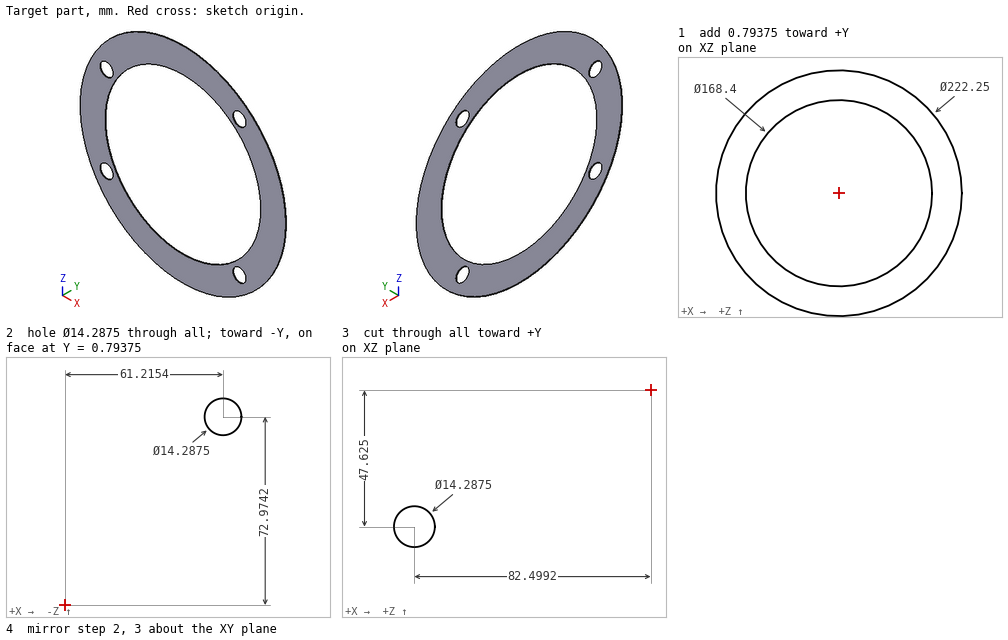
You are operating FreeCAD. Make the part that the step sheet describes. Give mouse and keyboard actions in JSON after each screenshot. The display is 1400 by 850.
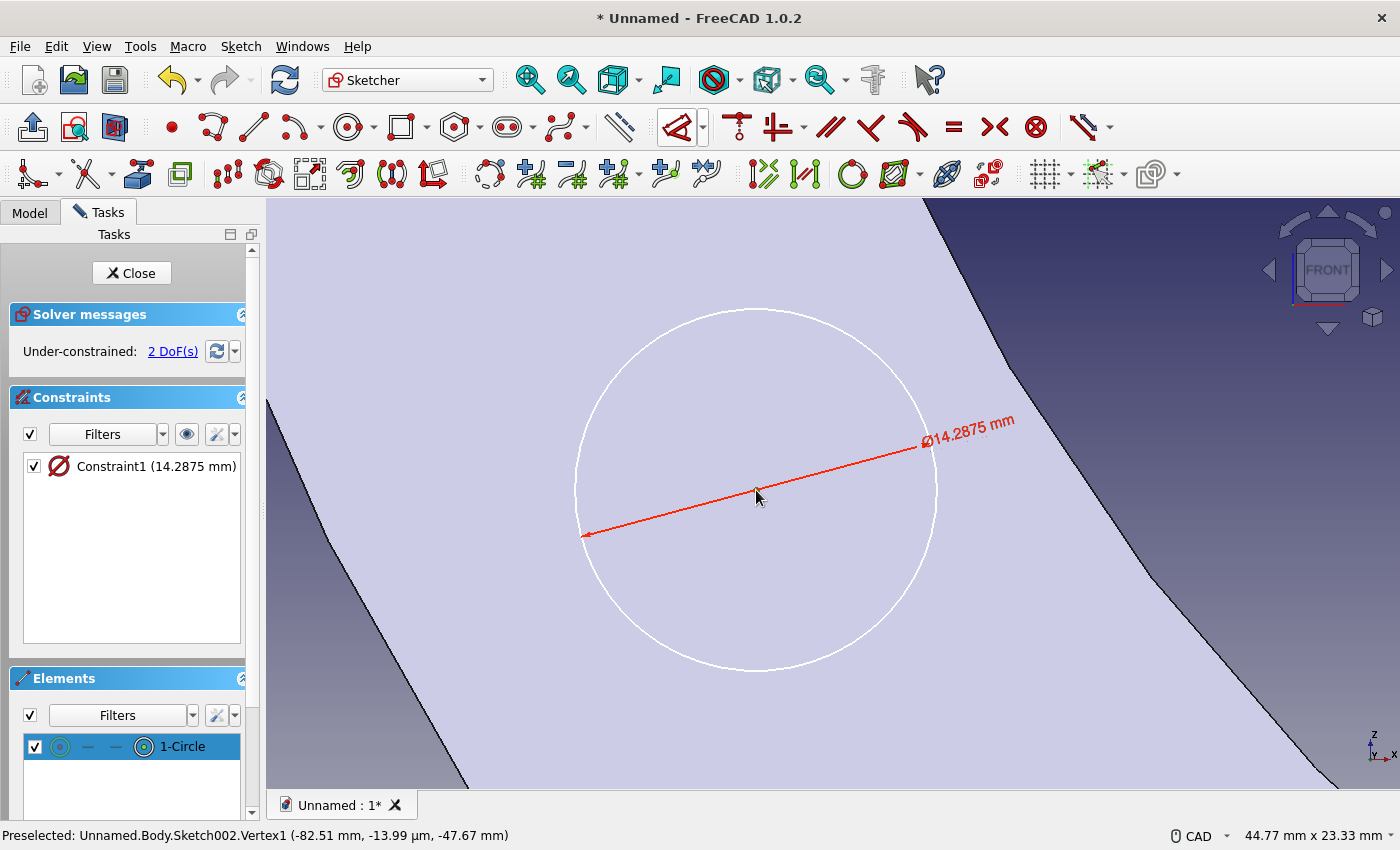
{"action": "left_click", "coordinate": [702, 128]}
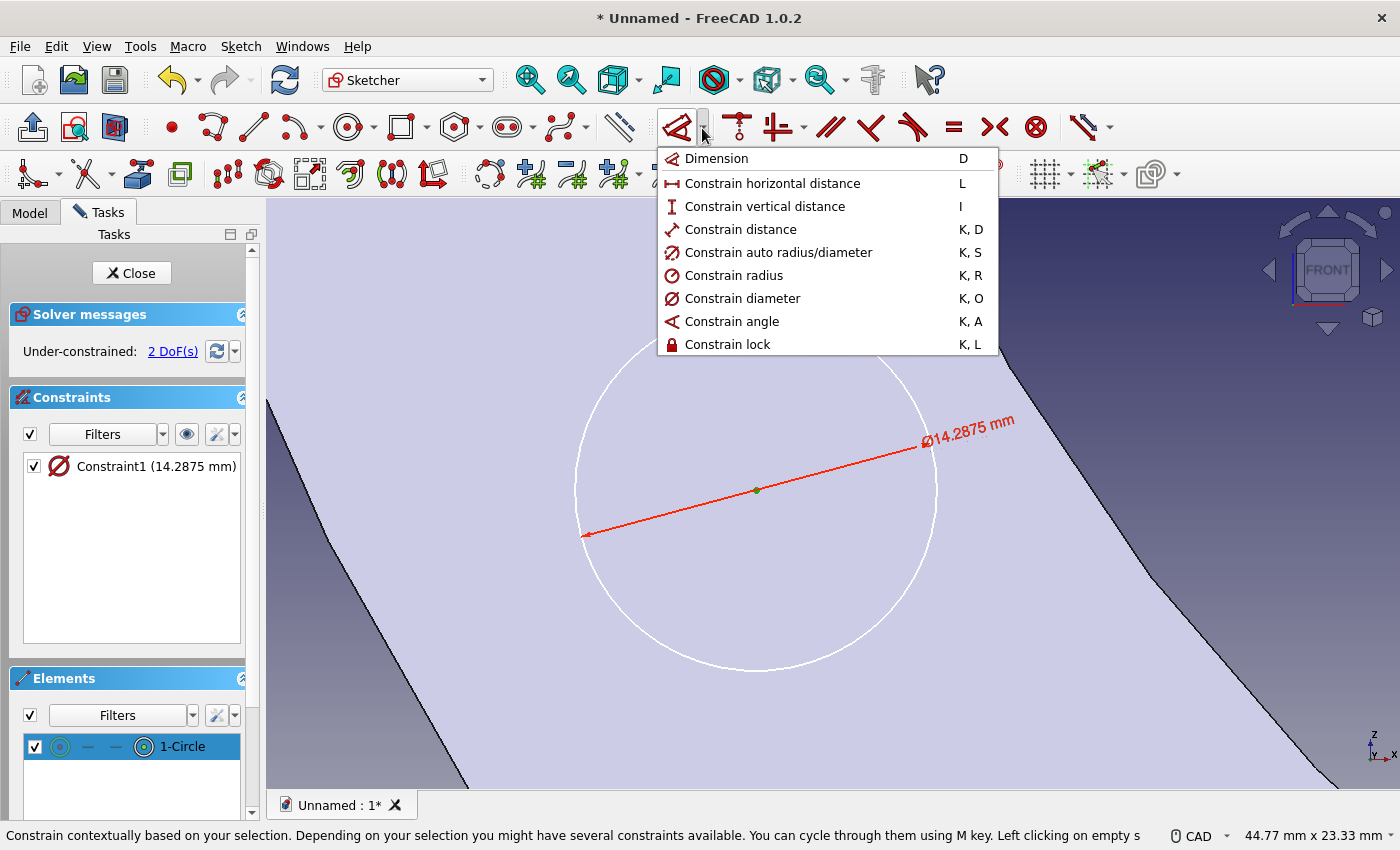
{"action": "left_click", "coordinate": [828, 206]}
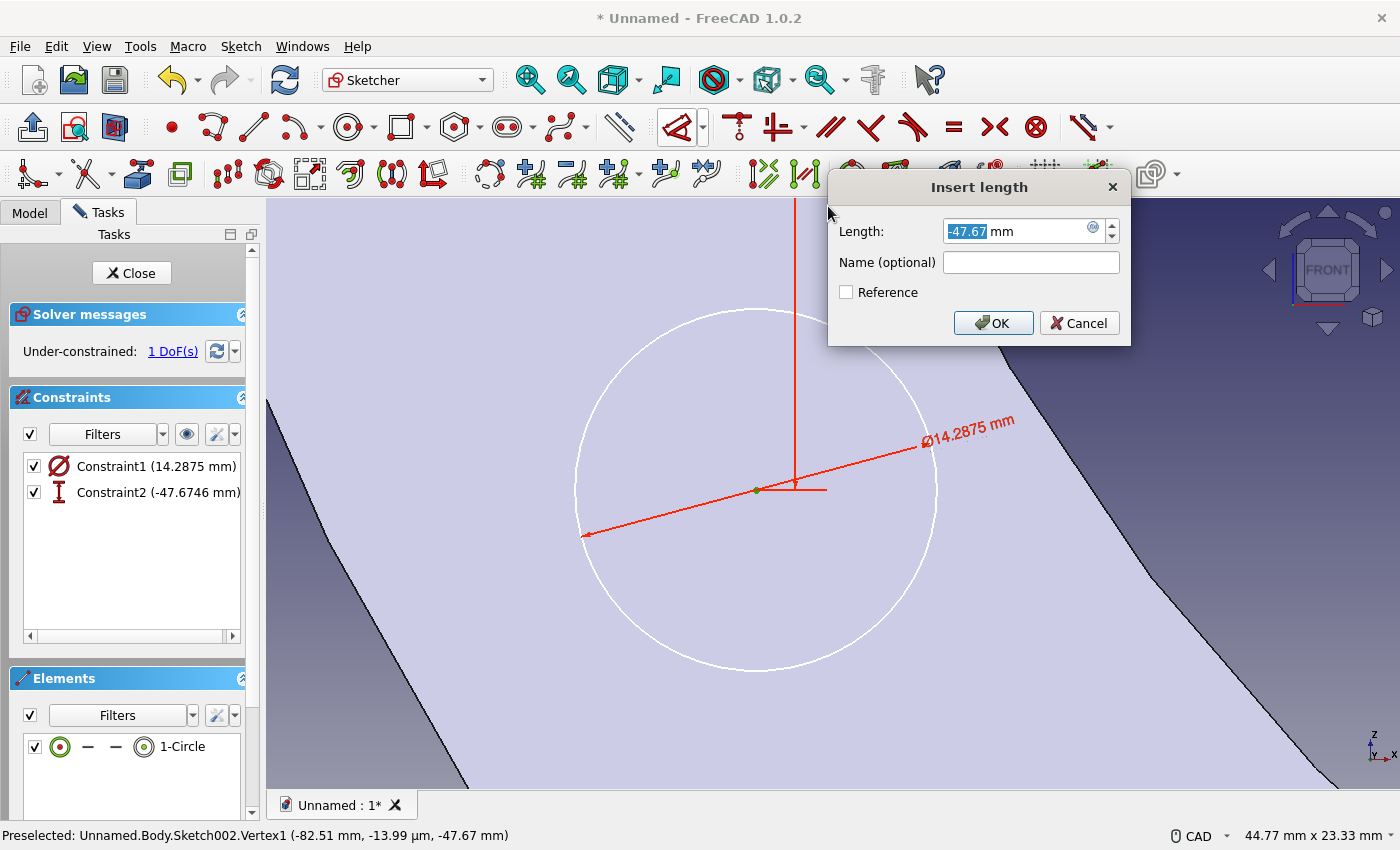
{"action": "type", "text": "-47.625"}
{"action": "key", "text": "Return"}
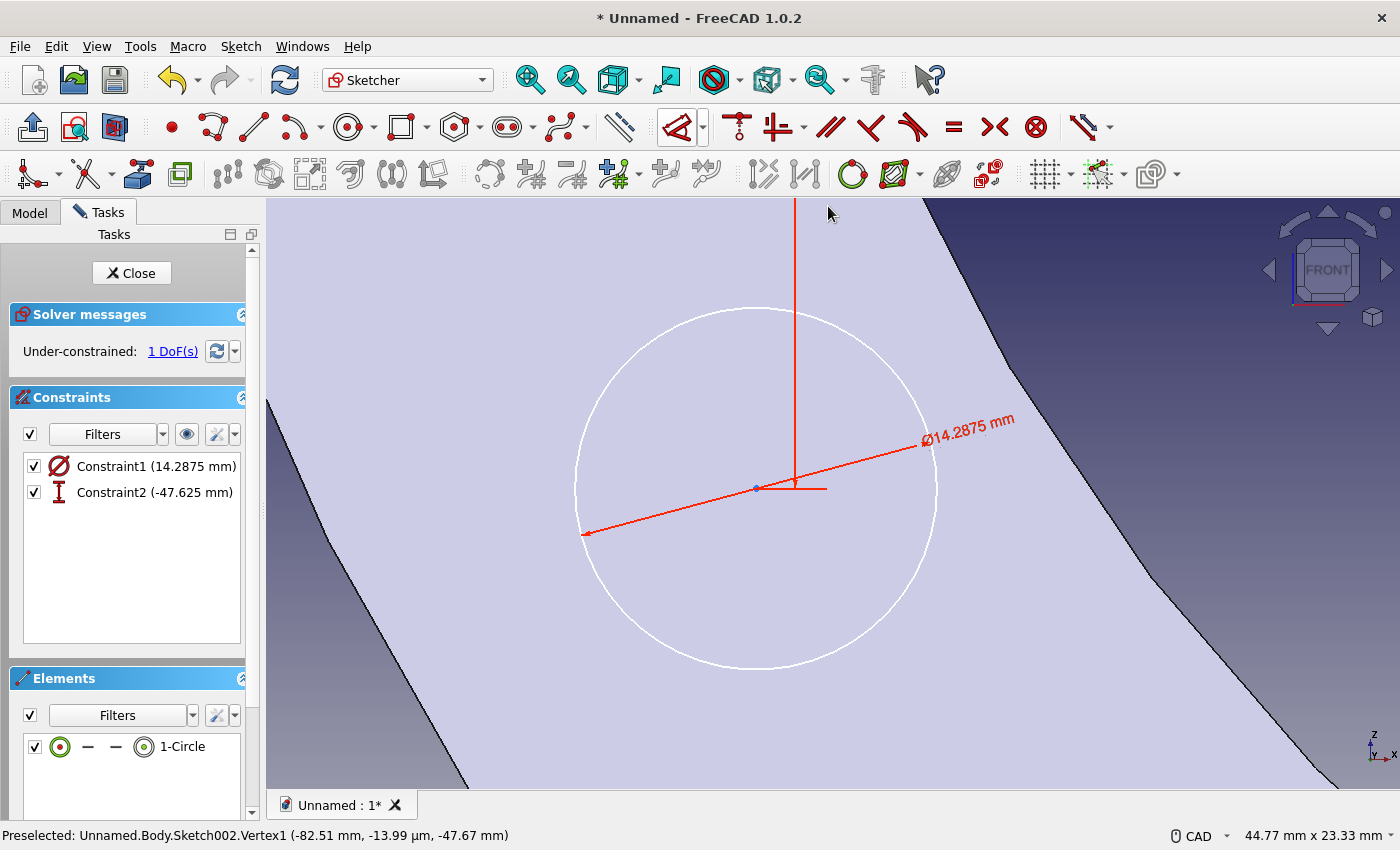
{"action": "left_click", "coordinate": [756, 489]}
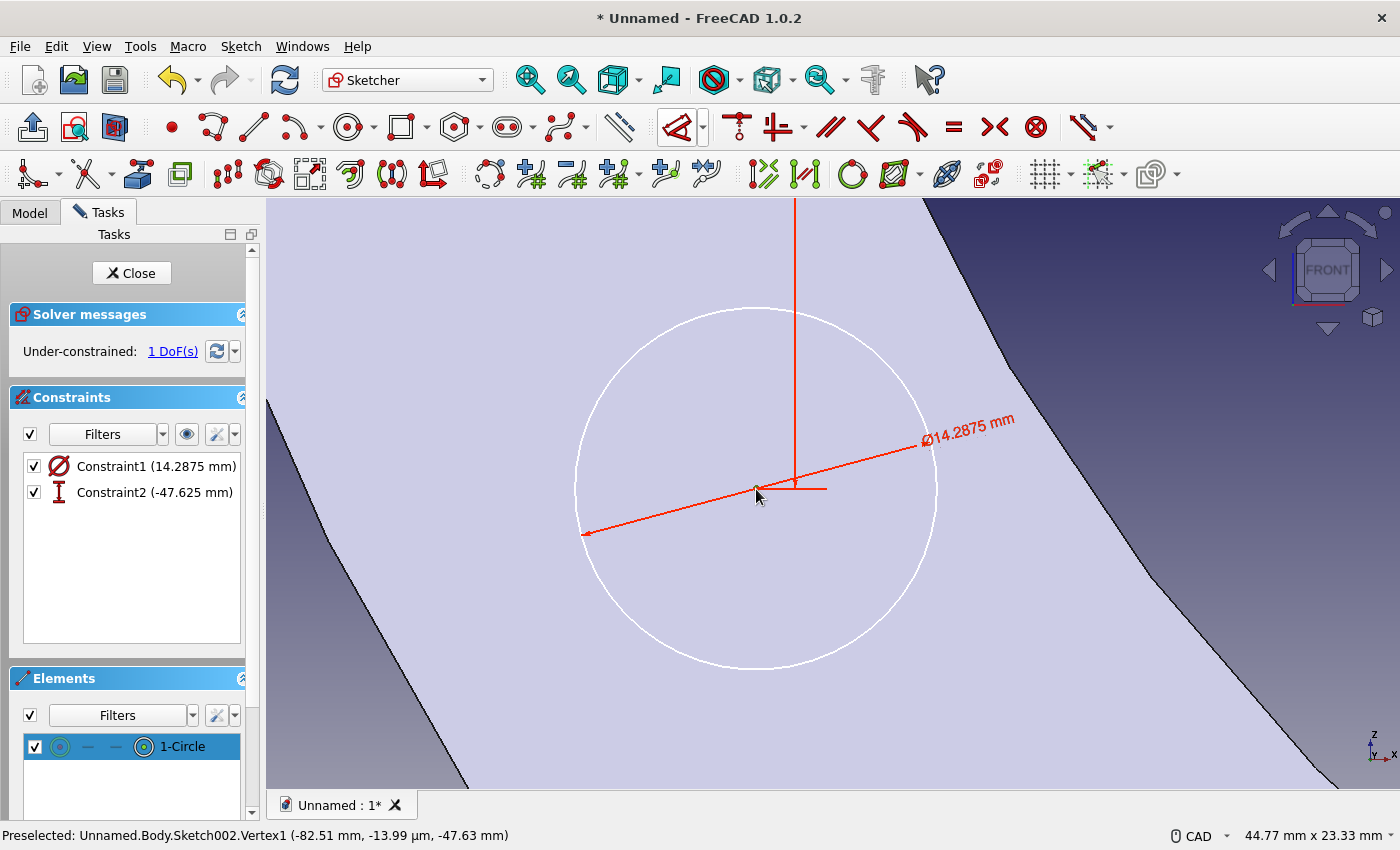
{"action": "left_click", "coordinate": [702, 128]}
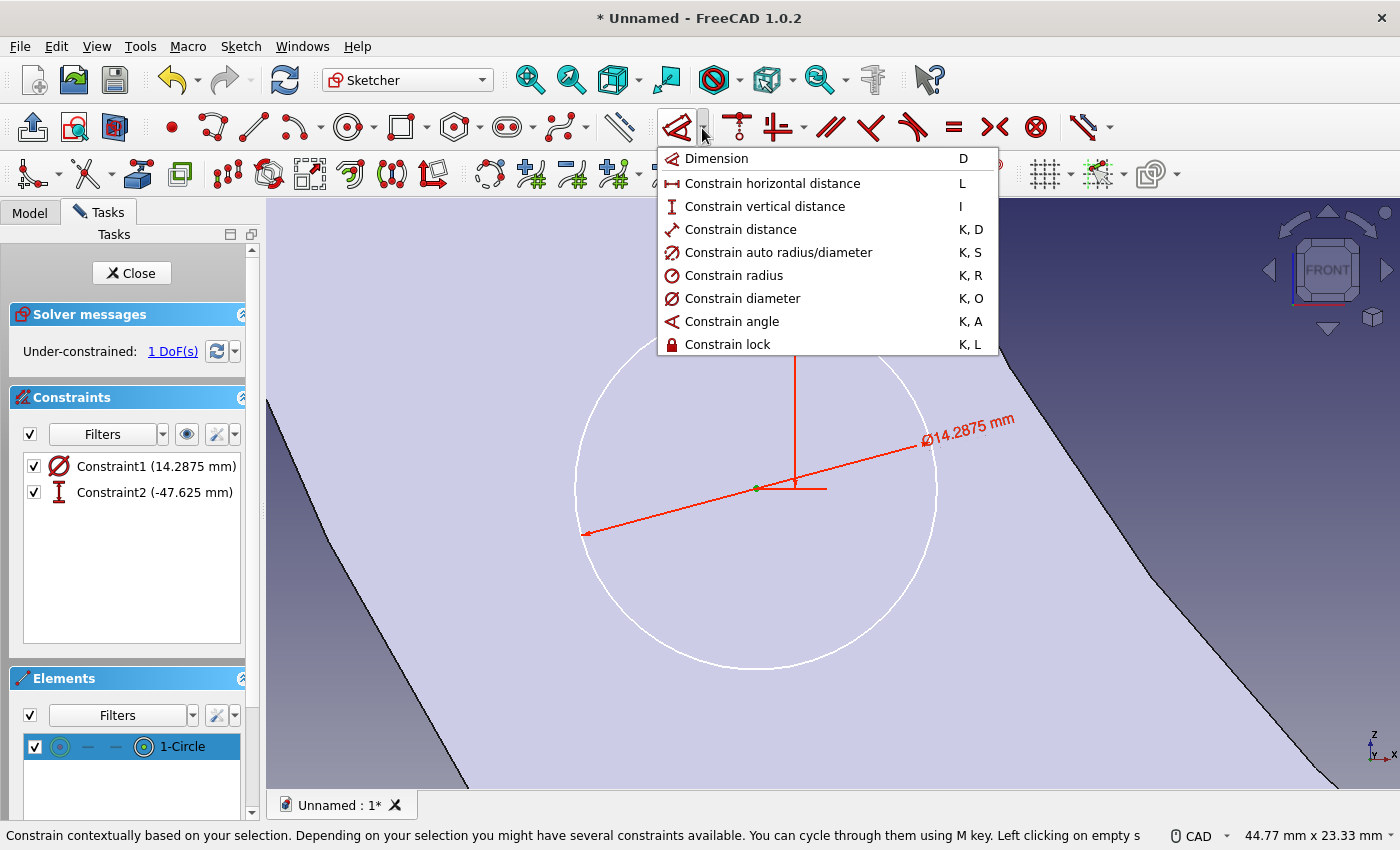
{"action": "left_click", "coordinate": [828, 184]}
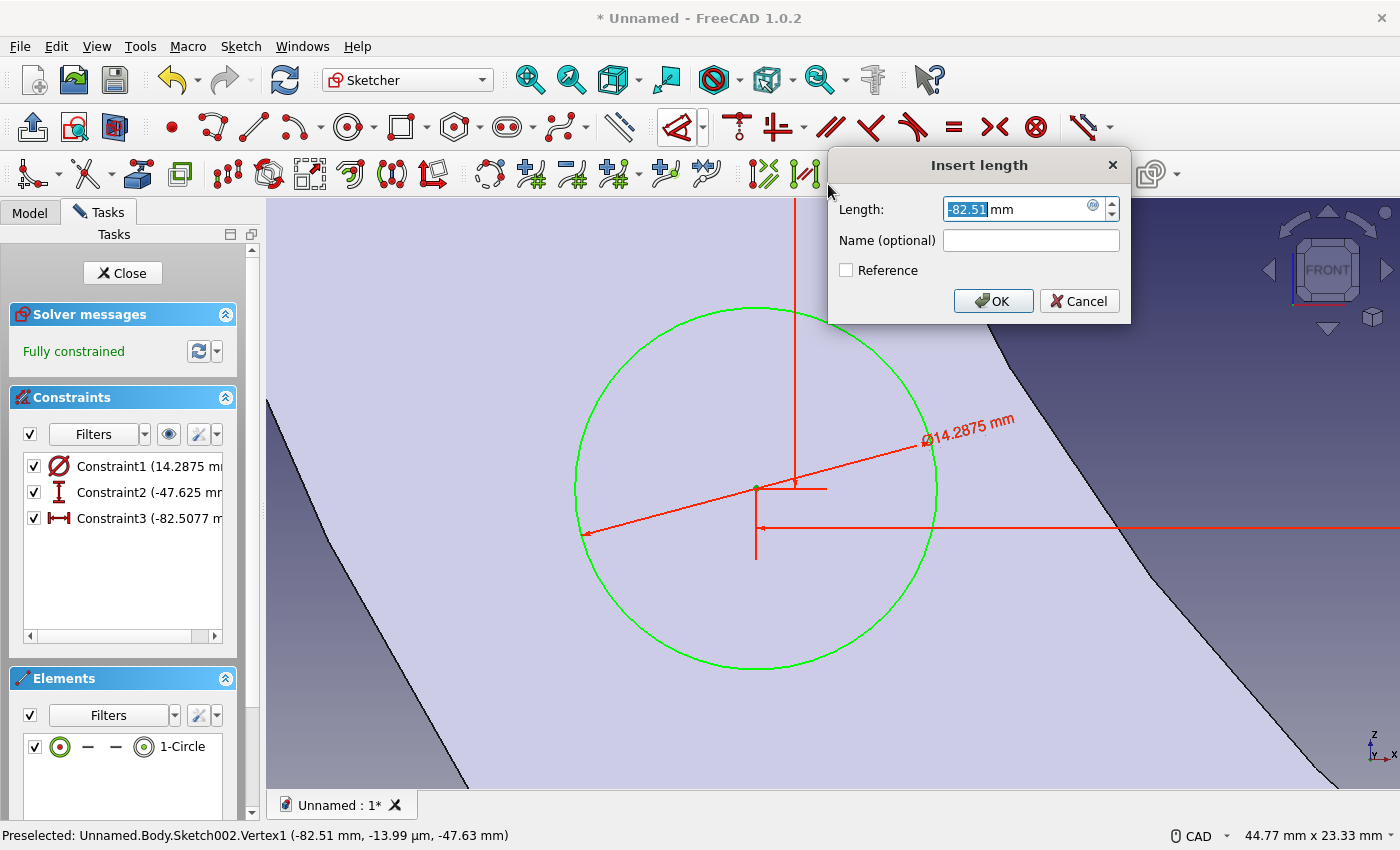
{"action": "type", "text": "-82.4992"}
{"action": "key", "text": "Return"}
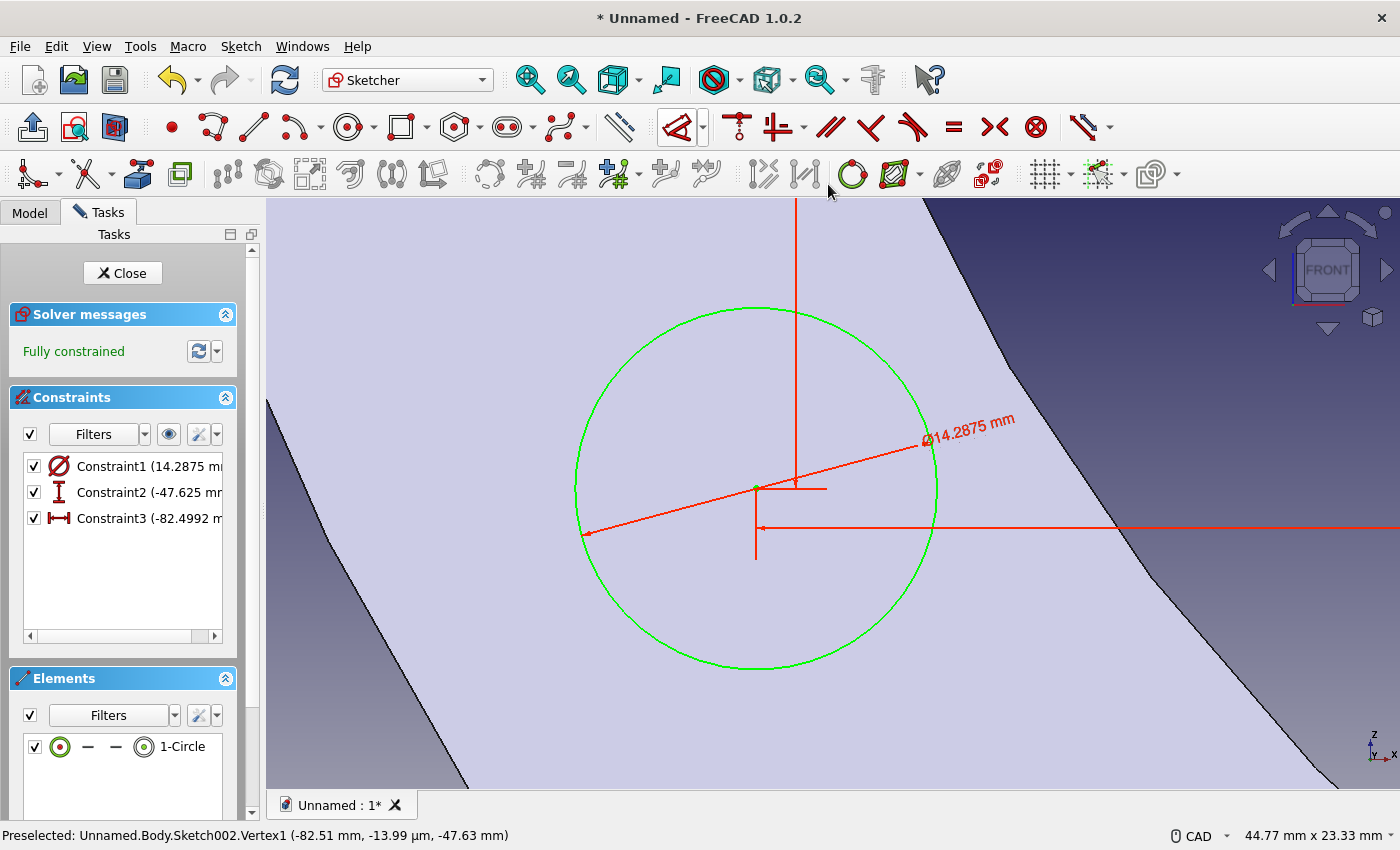
{"action": "left_click", "coordinate": [123, 273]}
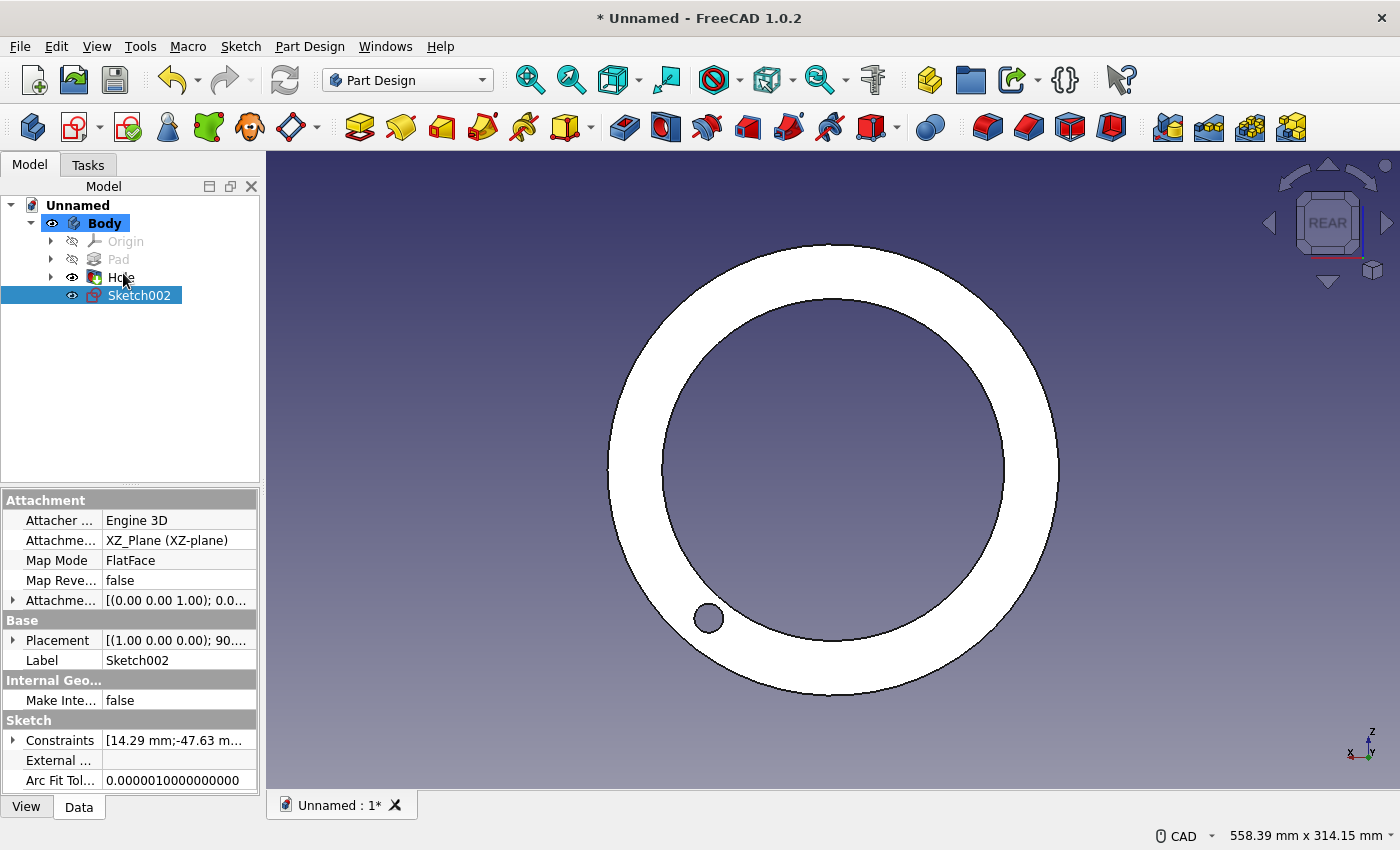
{"action": "left_click", "coordinate": [625, 128]}